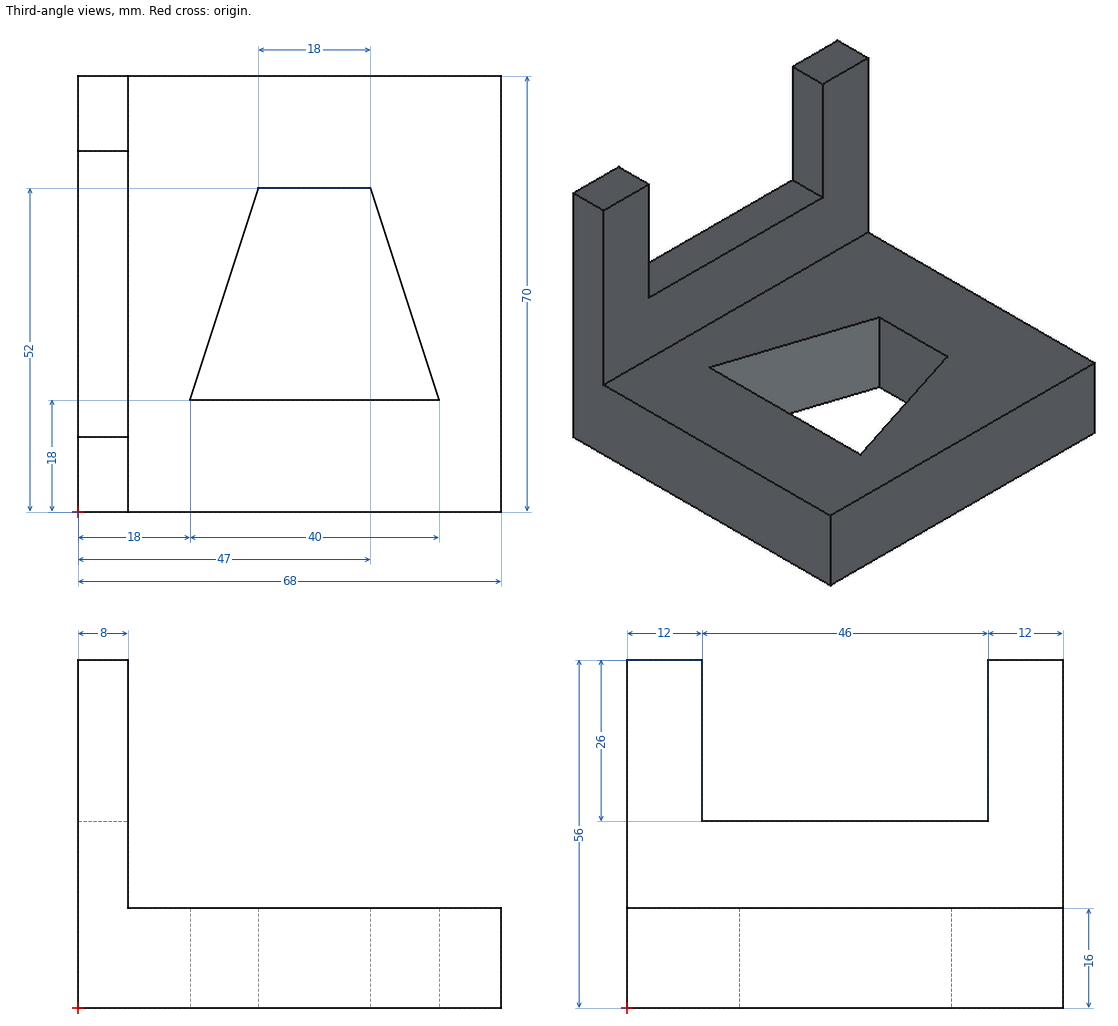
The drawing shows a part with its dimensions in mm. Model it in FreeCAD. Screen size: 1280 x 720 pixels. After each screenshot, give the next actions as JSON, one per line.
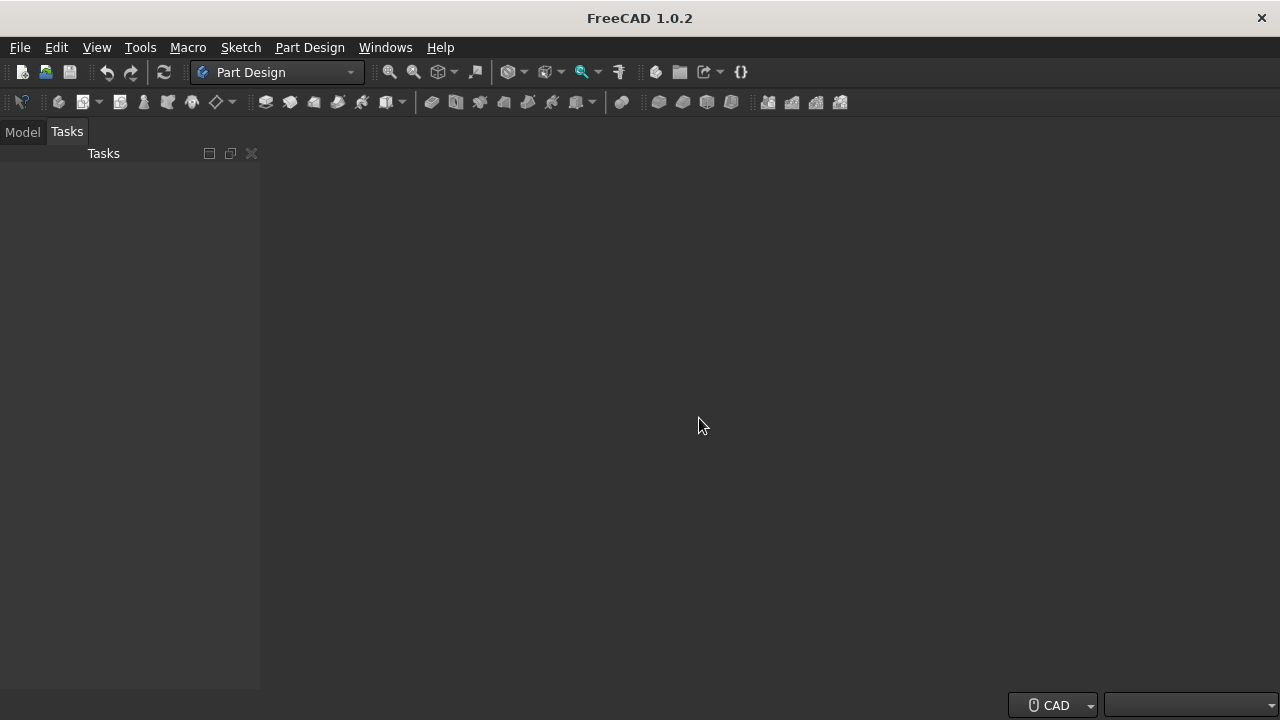
{"action": "left_click", "coordinate": [22, 72]}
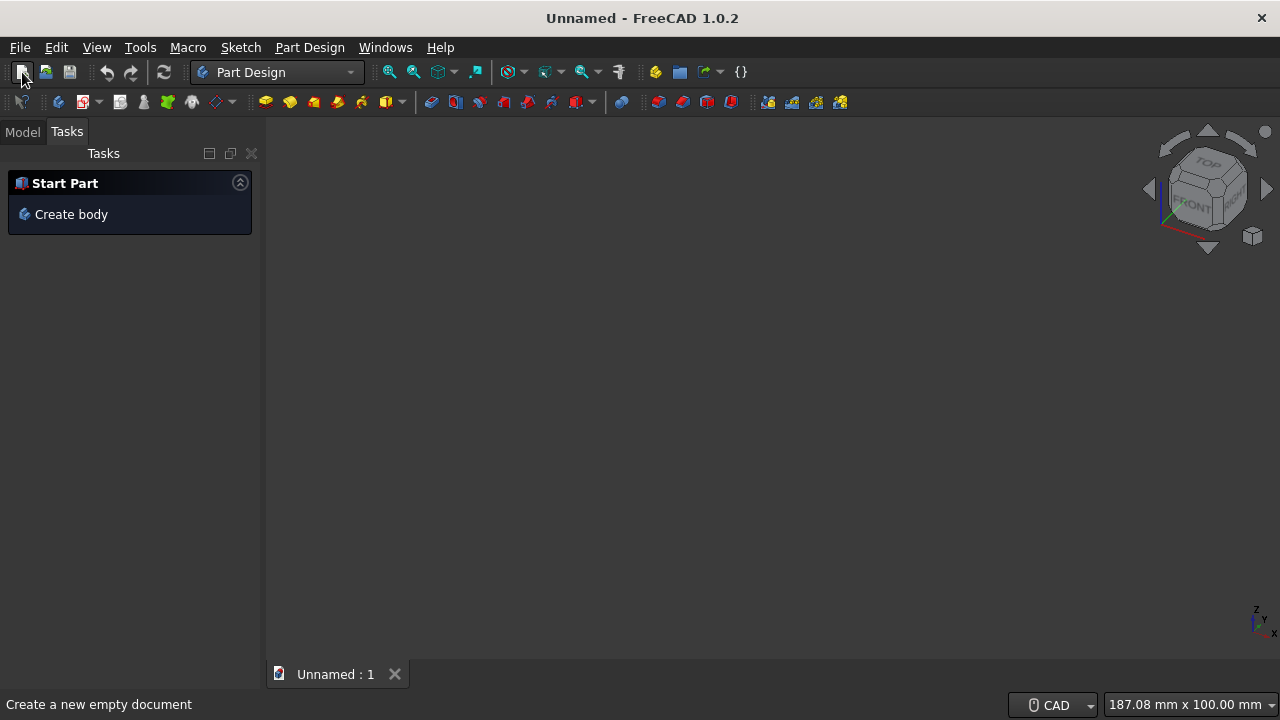
{"action": "left_click", "coordinate": [84, 102]}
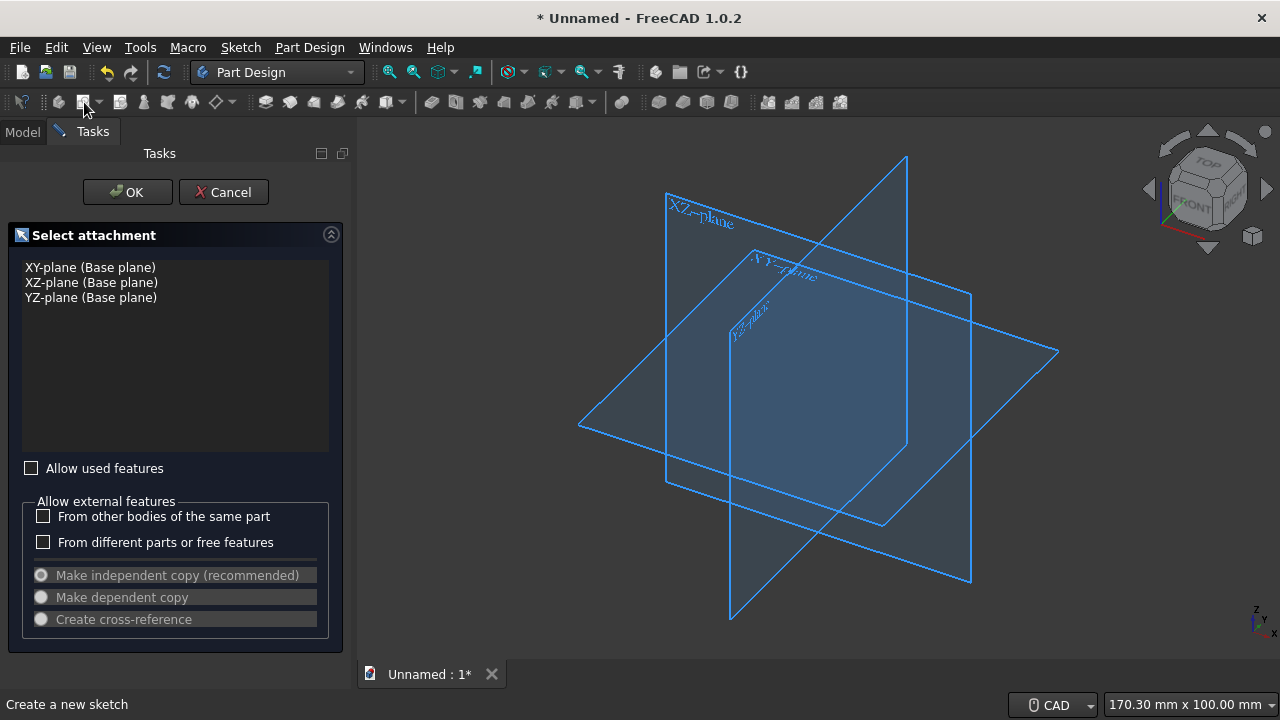
{"action": "left_click", "coordinate": [82, 268]}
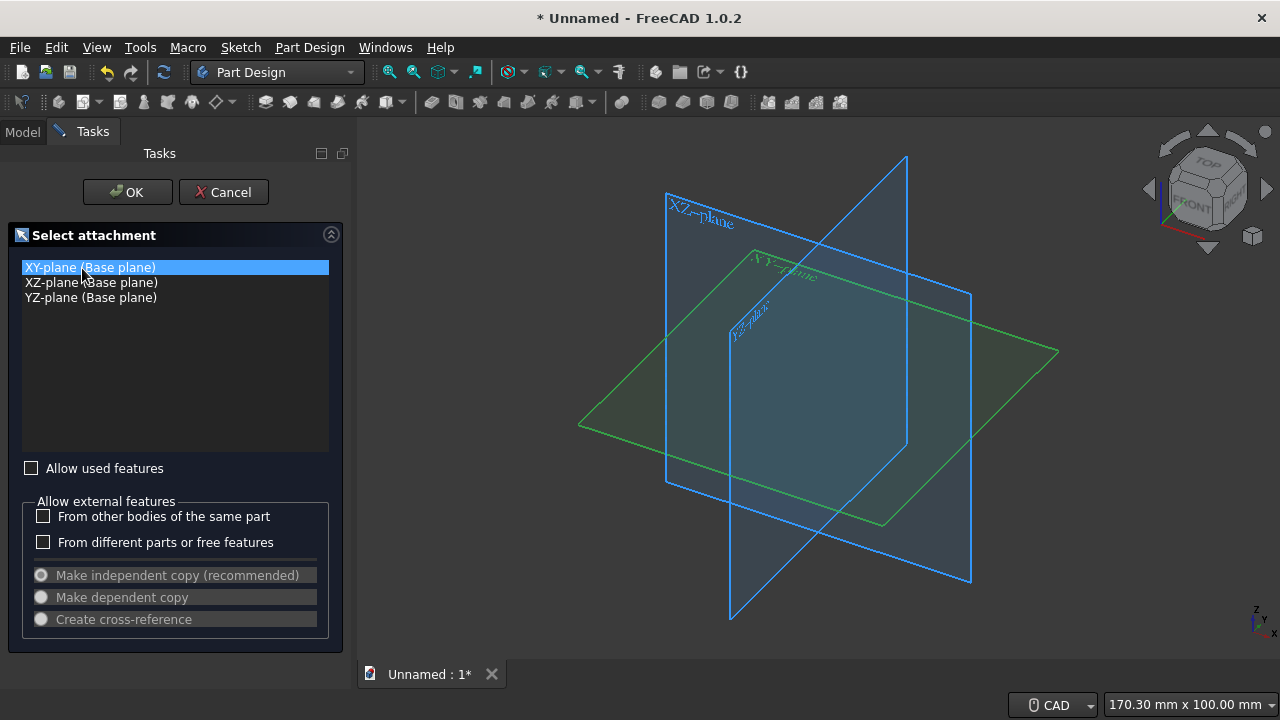
{"action": "left_click", "coordinate": [128, 192]}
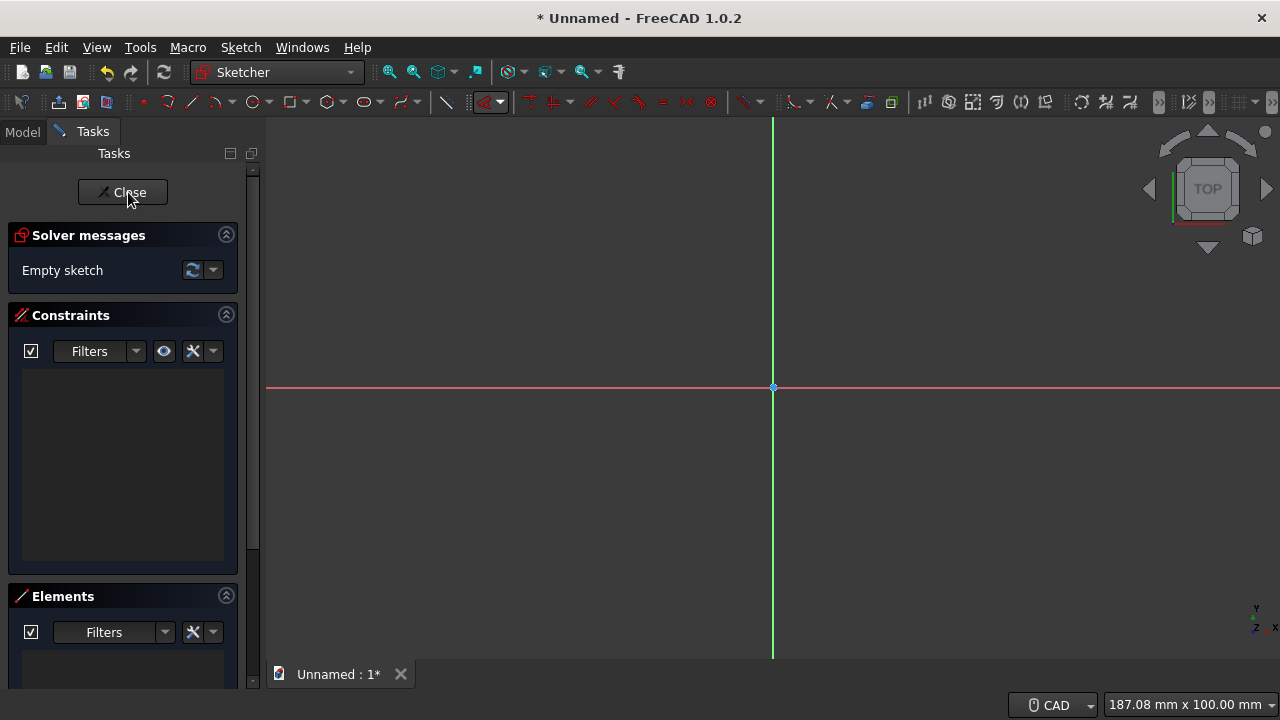
{"action": "scroll", "coordinate": [294, 631], "scroll_direction": "down", "scroll_amount": 2}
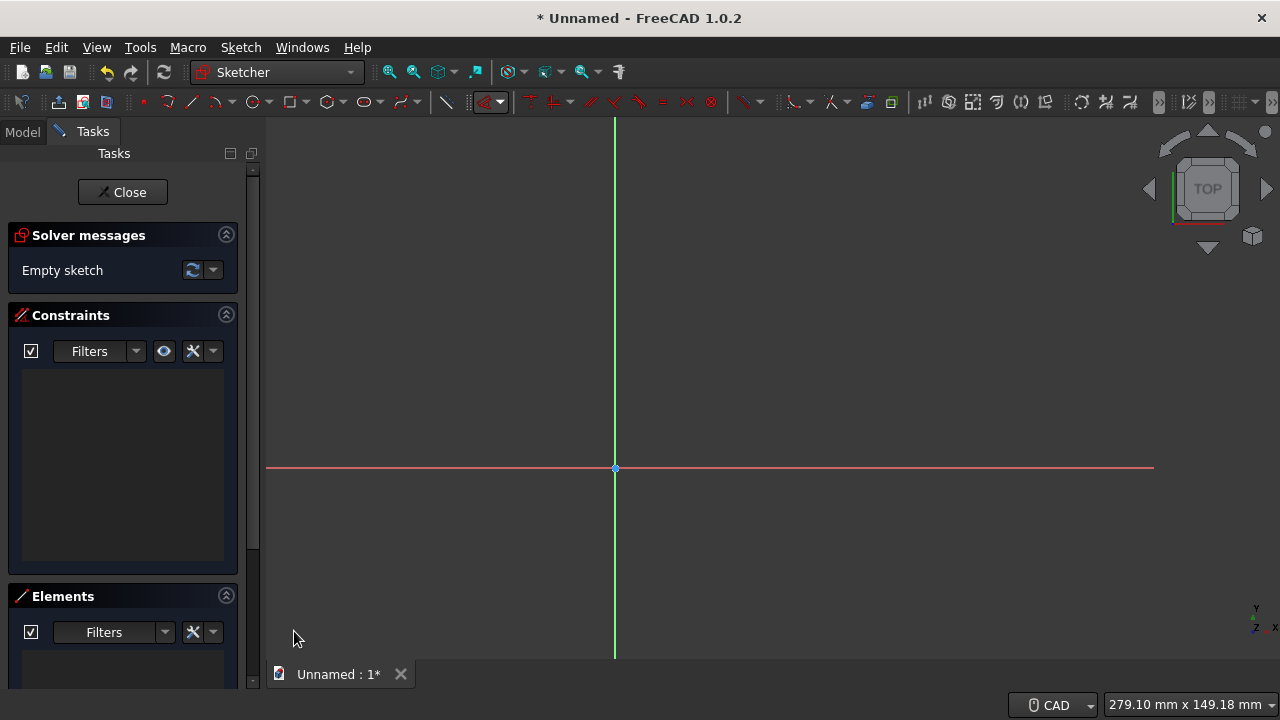
{"action": "left_click", "coordinate": [290, 102]}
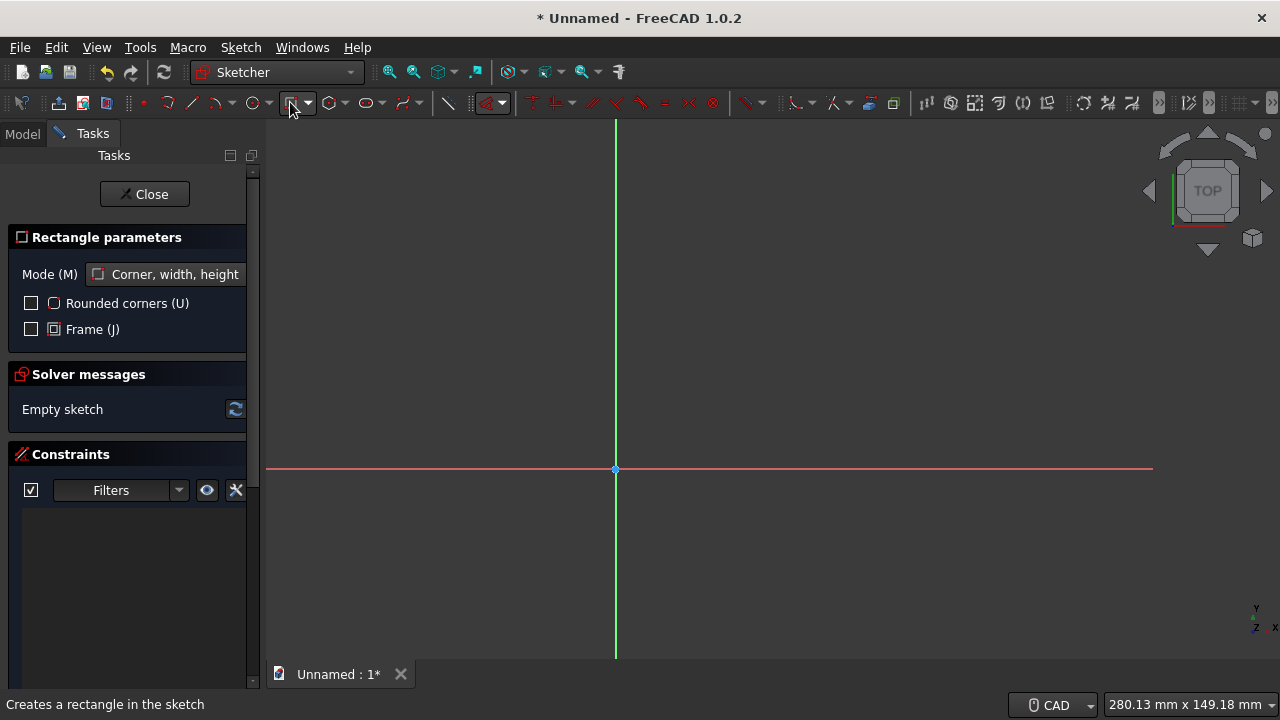
{"action": "left_click", "coordinate": [616, 469]}
{"action": "left_click", "coordinate": [862, 216]}
{"action": "key", "text": "Escape"}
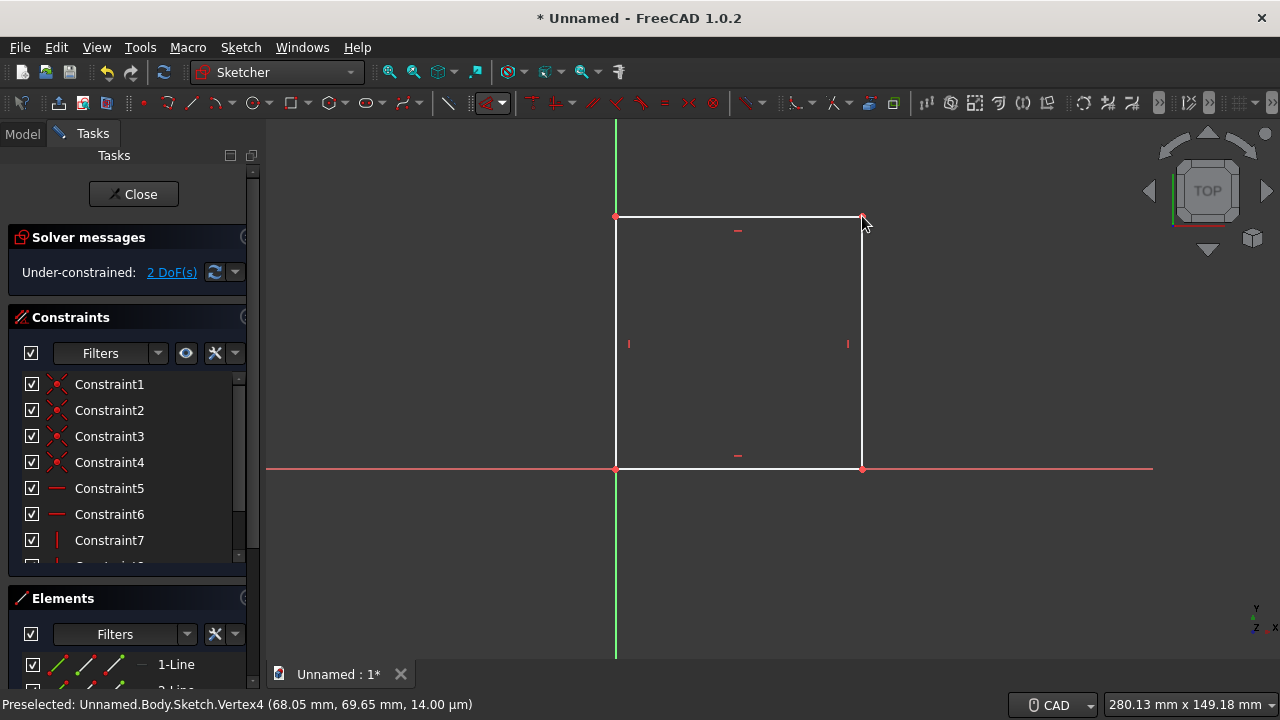
{"action": "left_click", "coordinate": [690, 469]}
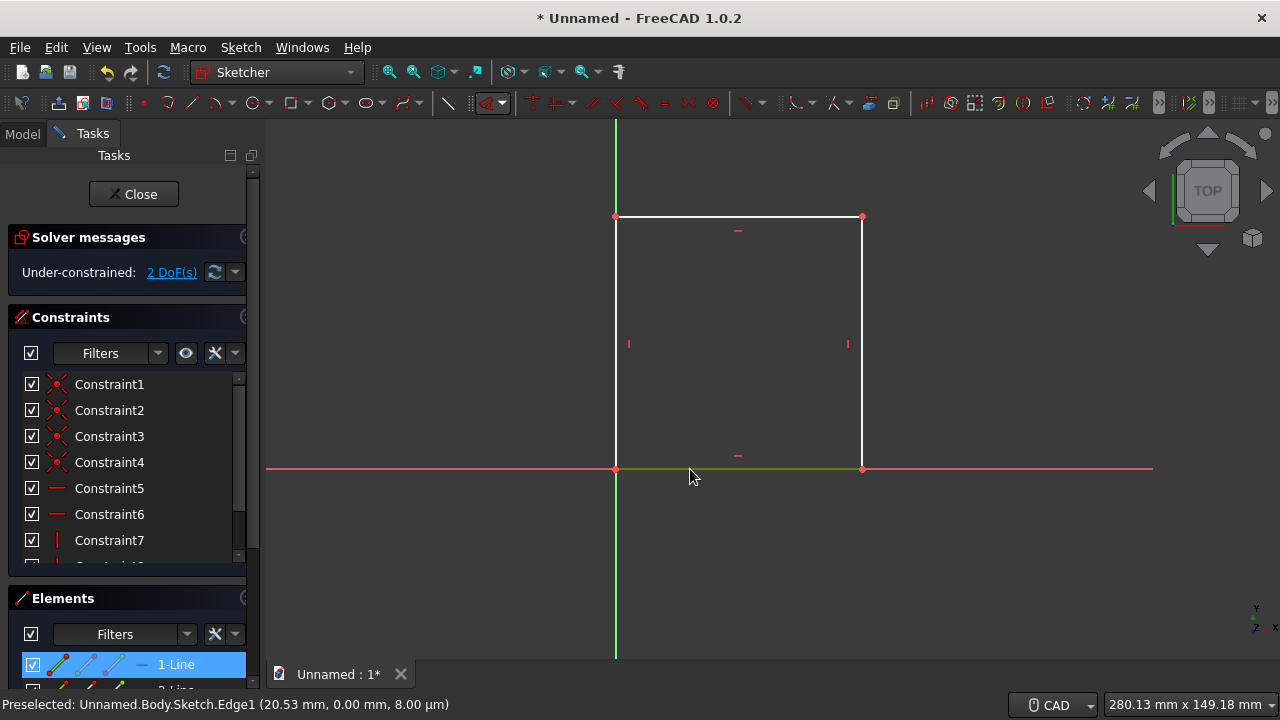
{"action": "key", "text": "l"}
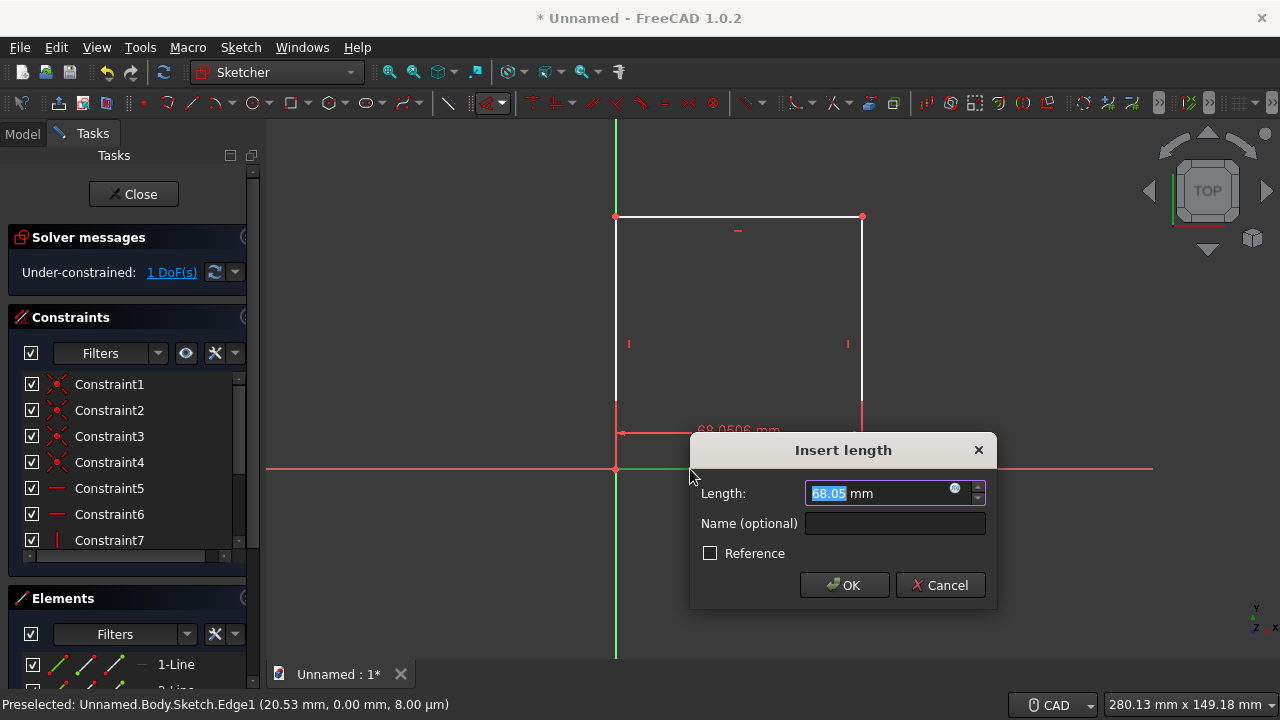
{"action": "type", "text": "68"}
{"action": "key", "text": "Return"}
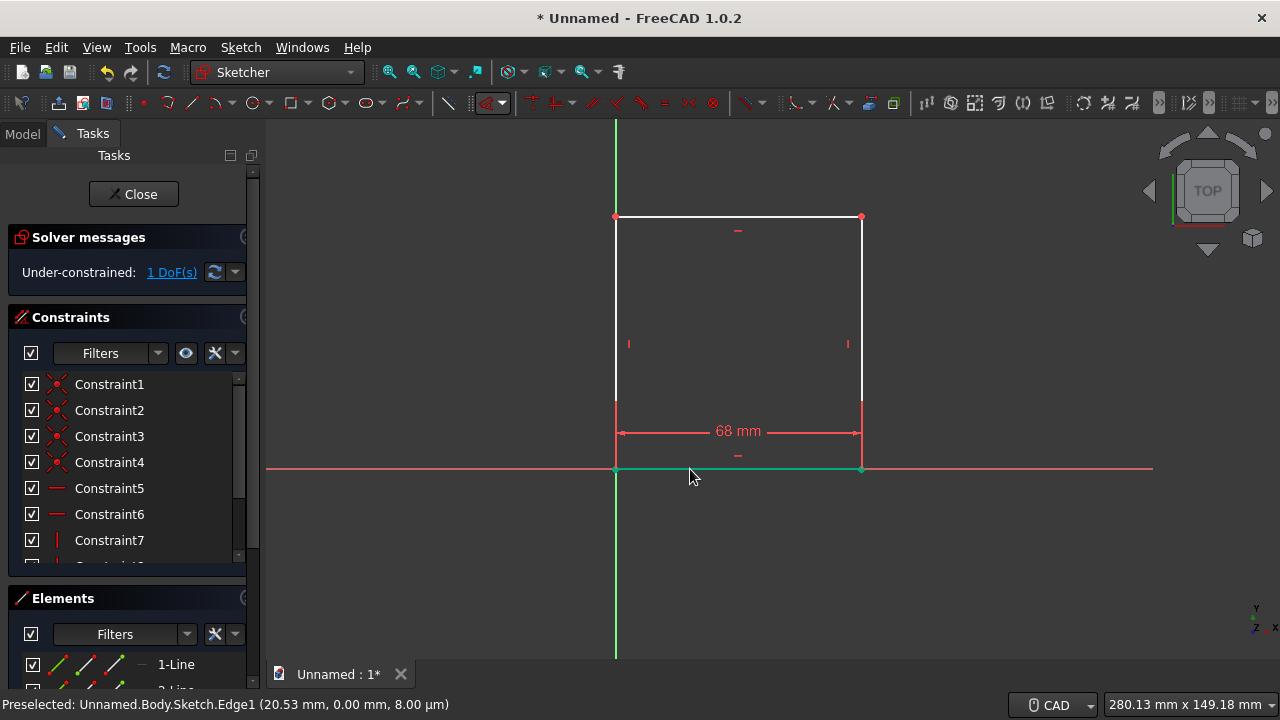
{"action": "left_click", "coordinate": [862, 393]}